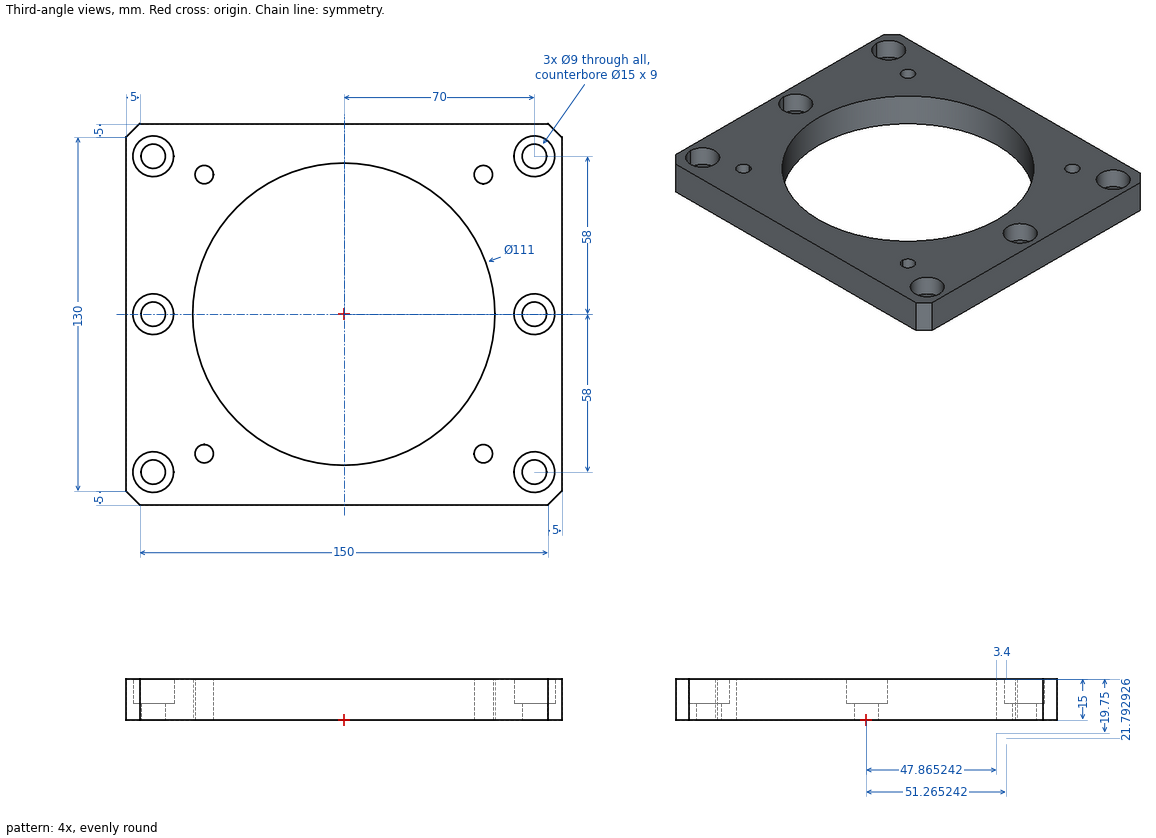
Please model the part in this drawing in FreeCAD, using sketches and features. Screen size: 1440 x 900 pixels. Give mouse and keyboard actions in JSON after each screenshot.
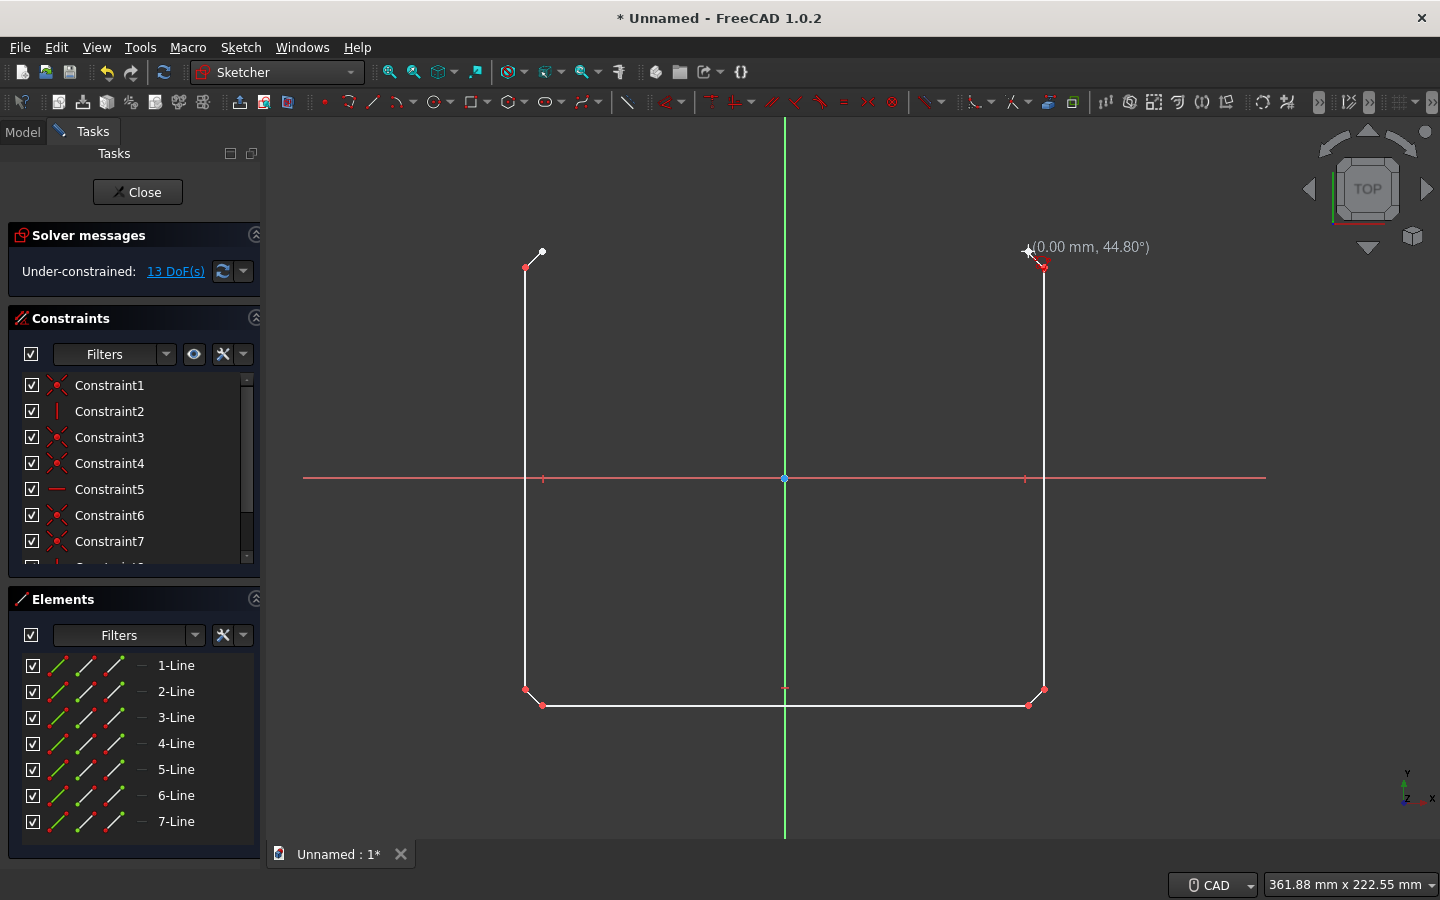
{"action": "scroll", "coordinate": [542, 251], "scroll_direction": "up", "scroll_amount": 2}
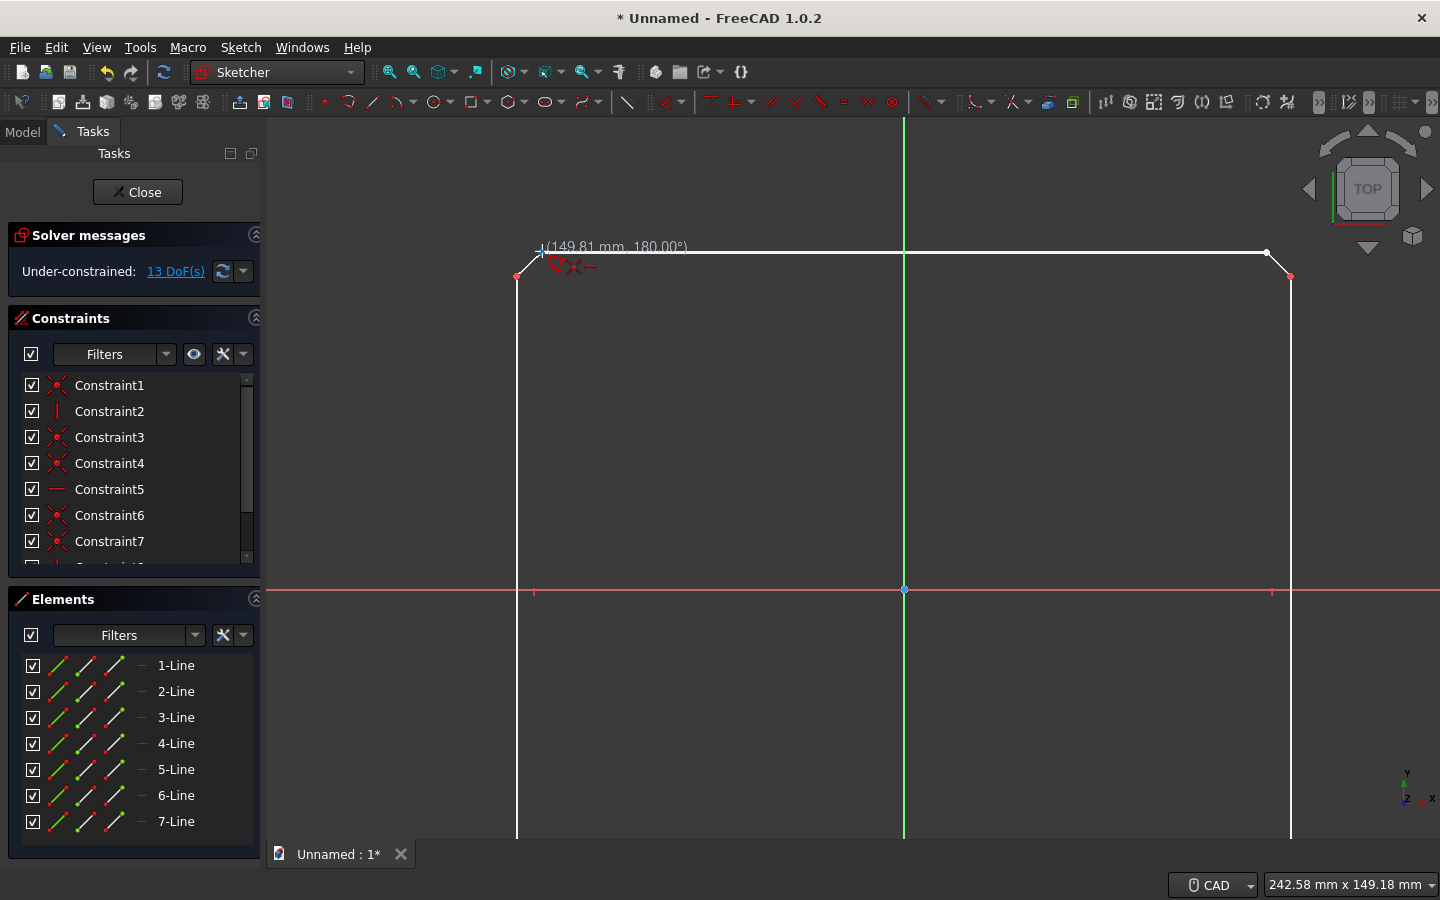
{"action": "left_click", "coordinate": [542, 252]}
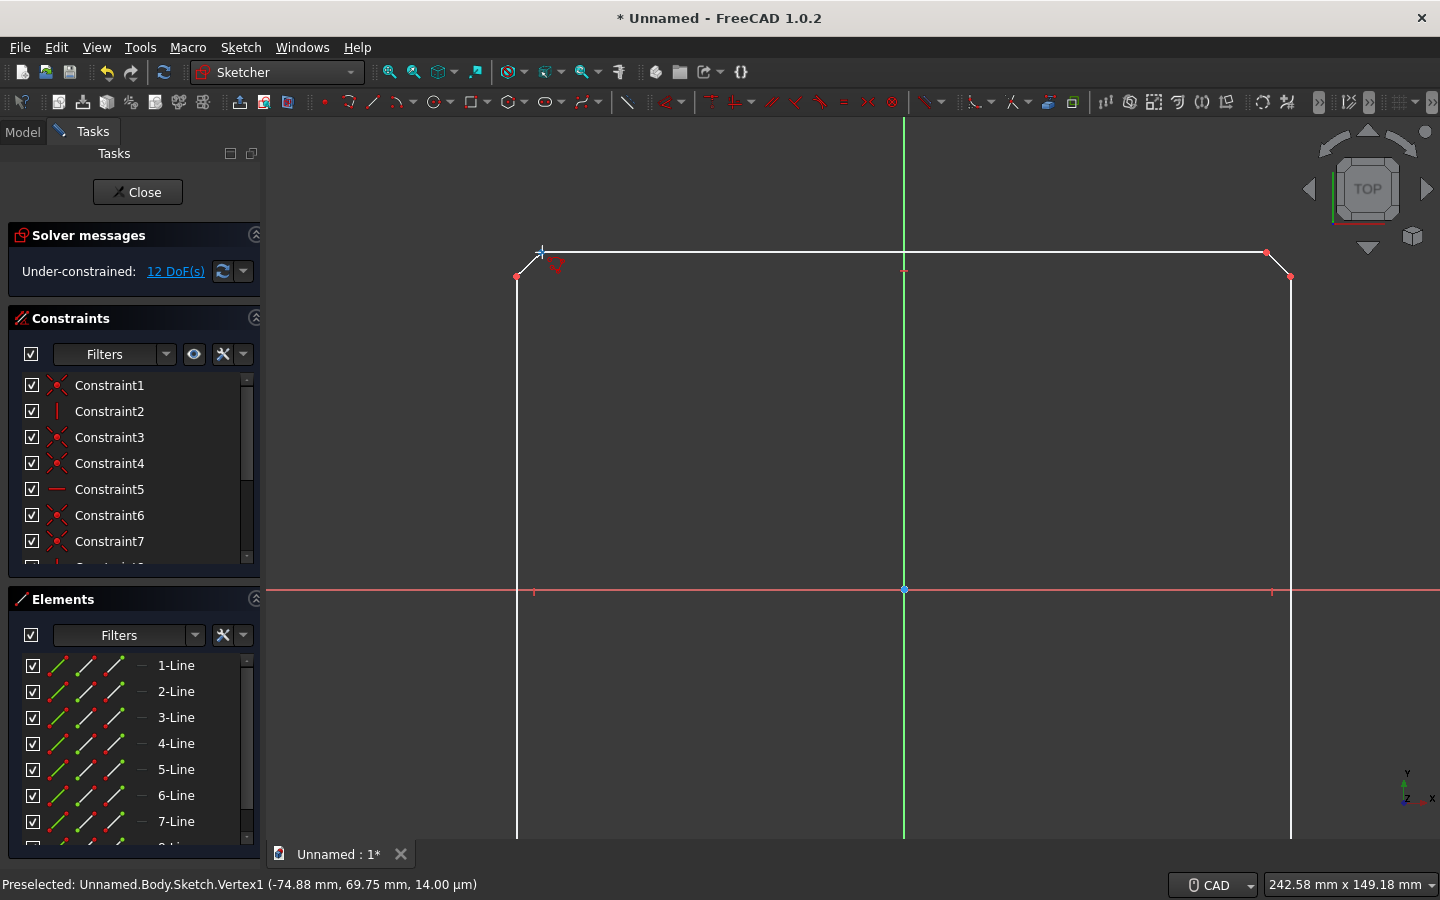
{"action": "left_click", "coordinate": [434, 102]}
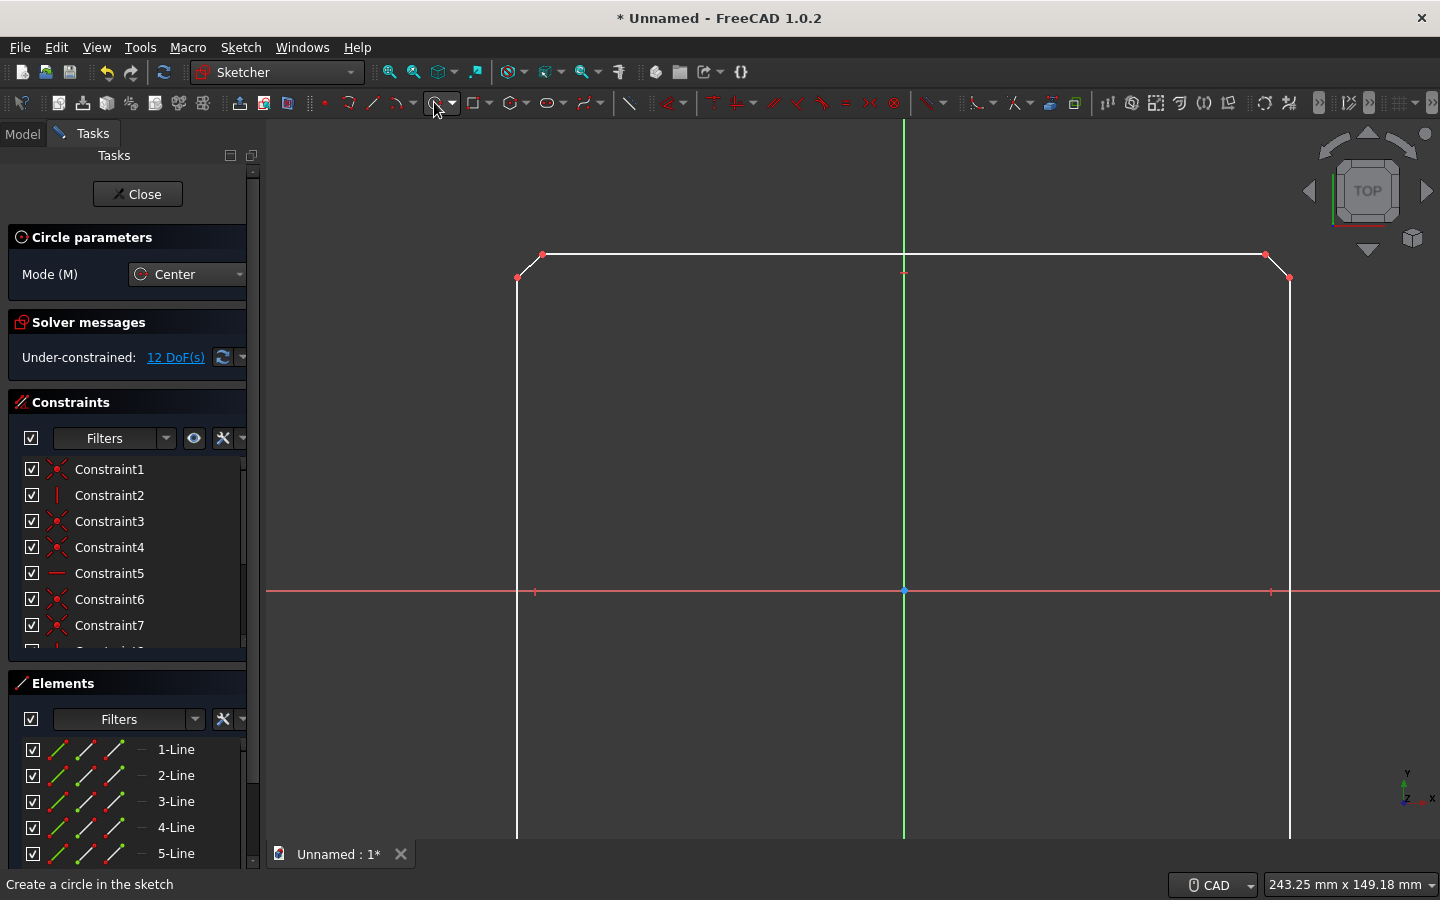
{"action": "left_click", "coordinate": [904, 591]}
{"action": "mouse_move", "coordinate": [1094, 401]}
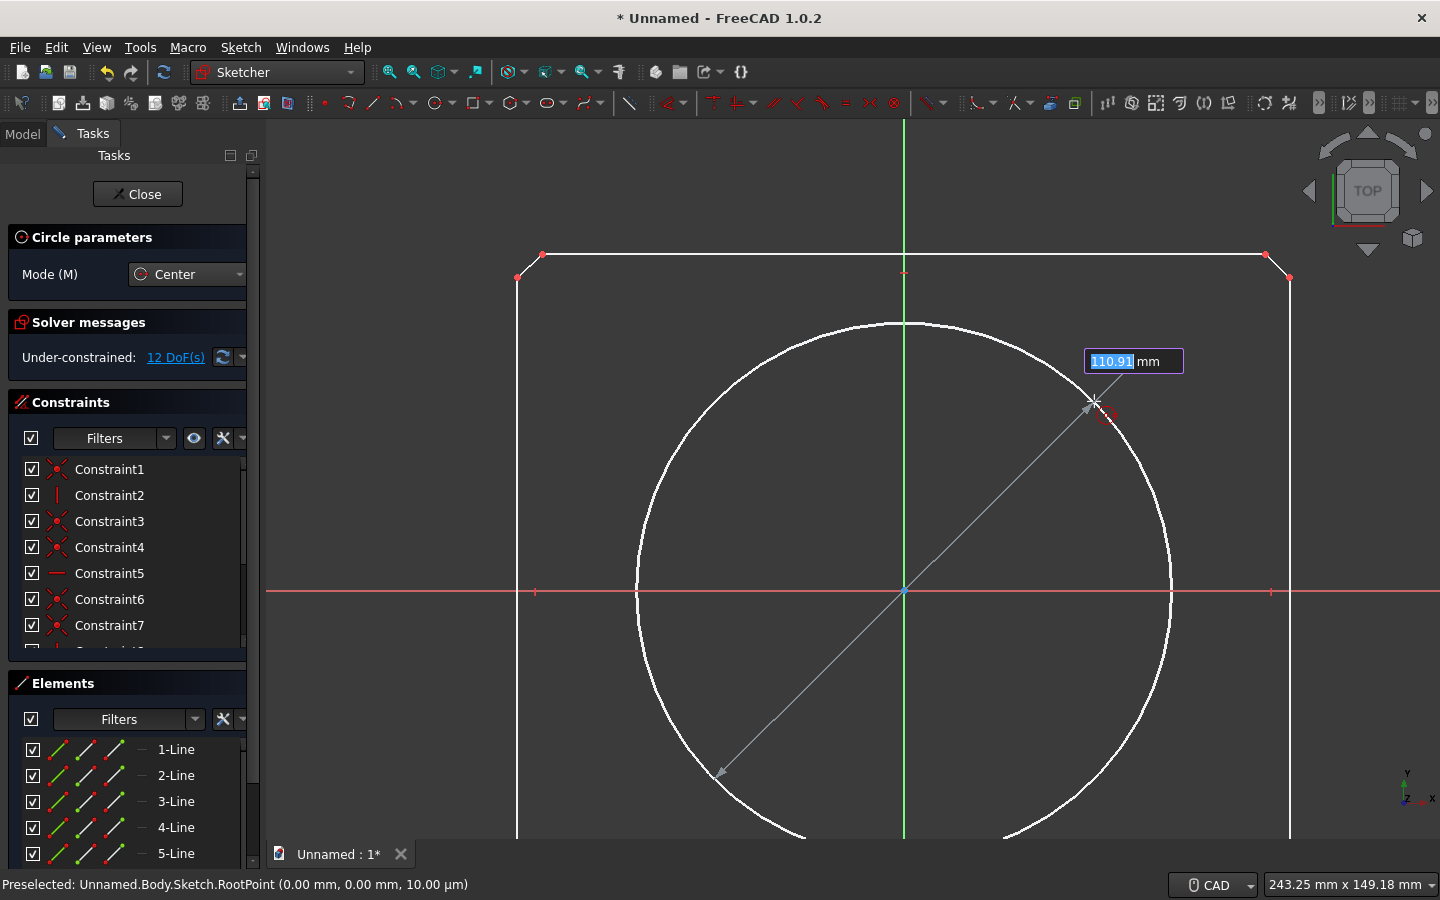
{"action": "type", "text": "111"}
{"action": "key", "text": "Return"}
{"action": "key", "text": "Escape"}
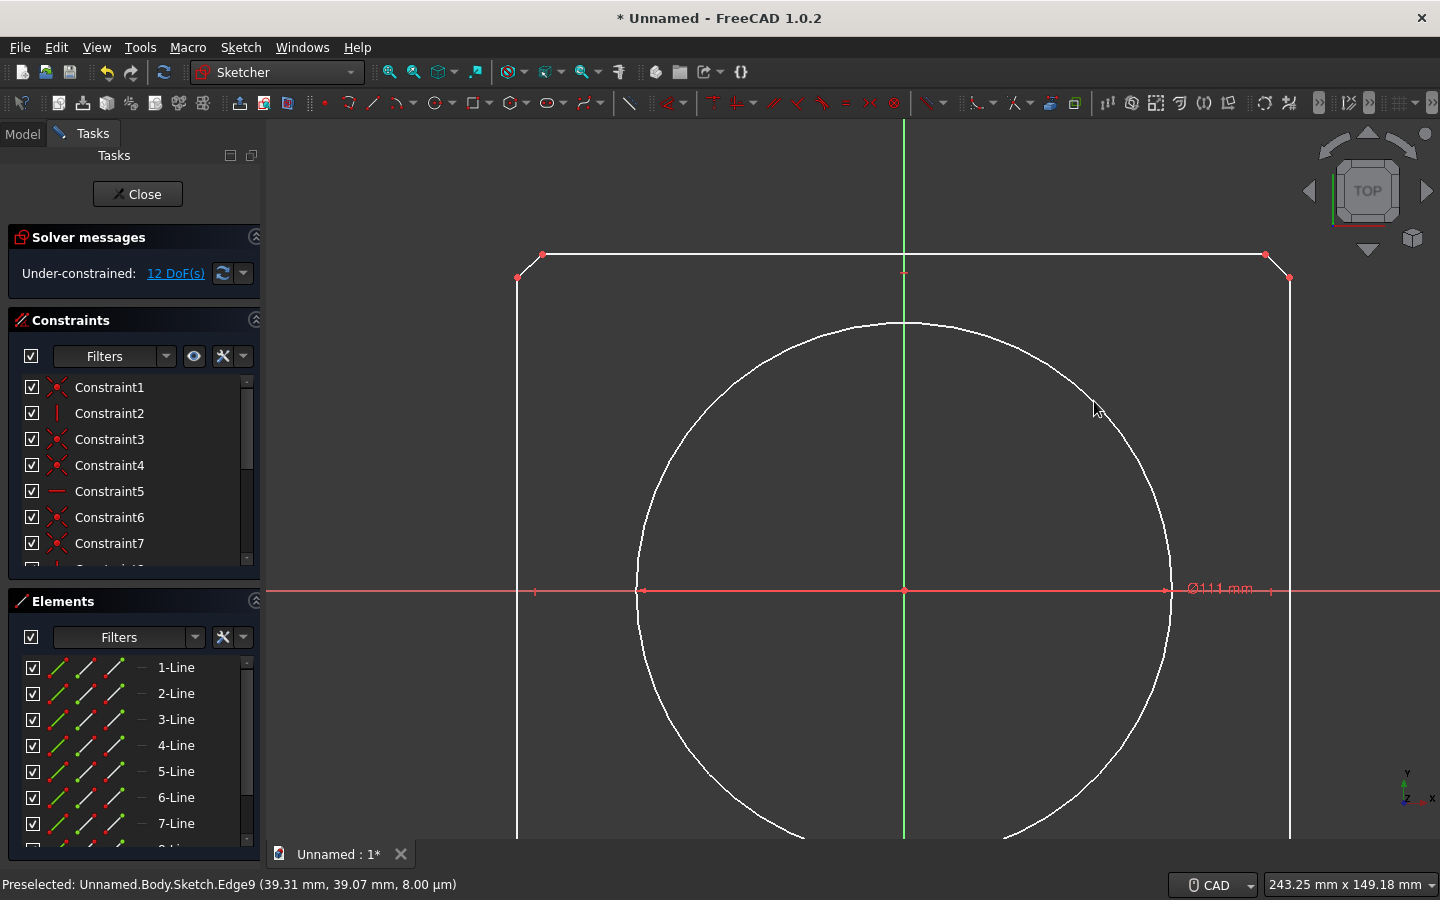
{"action": "left_click", "coordinate": [543, 254]}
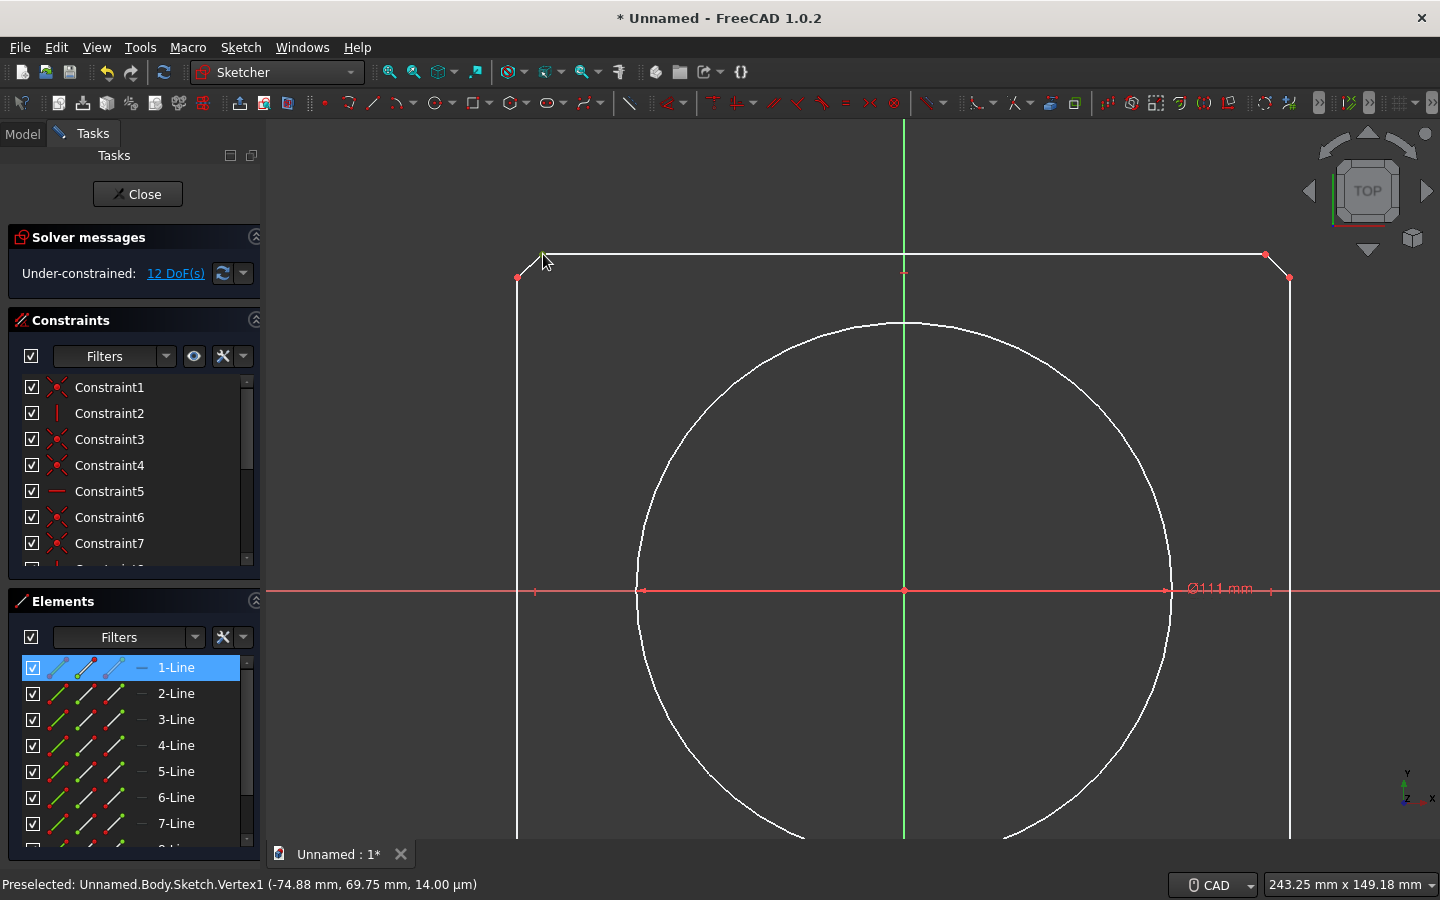
{"action": "scroll", "coordinate": [541, 252], "scroll_direction": "down", "scroll_amount": 2}